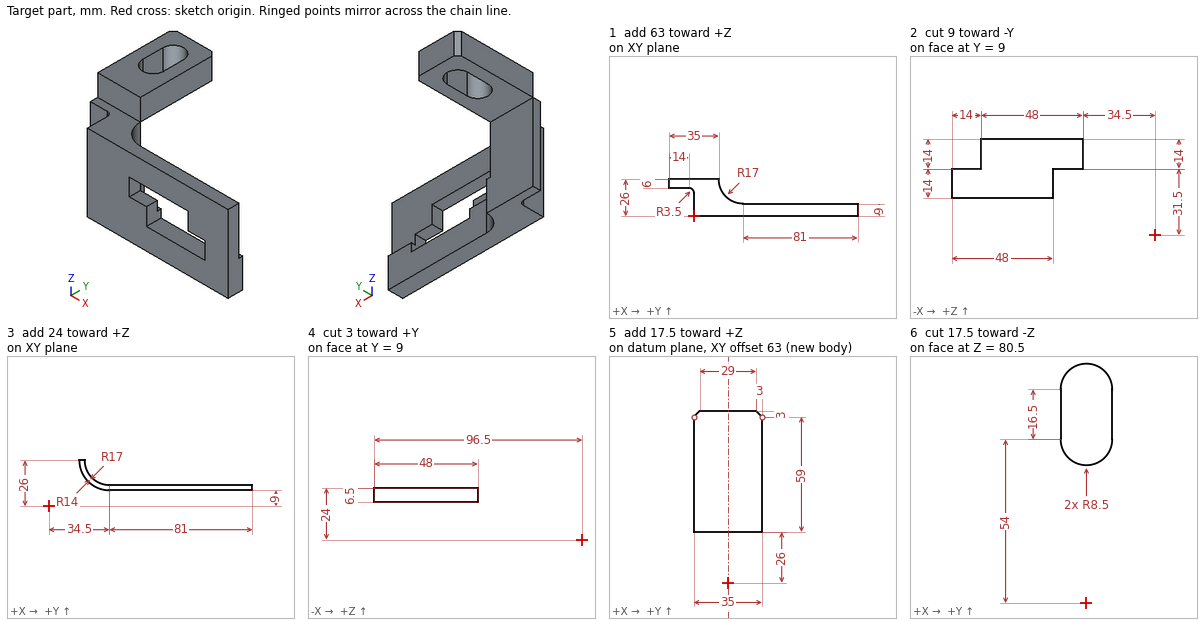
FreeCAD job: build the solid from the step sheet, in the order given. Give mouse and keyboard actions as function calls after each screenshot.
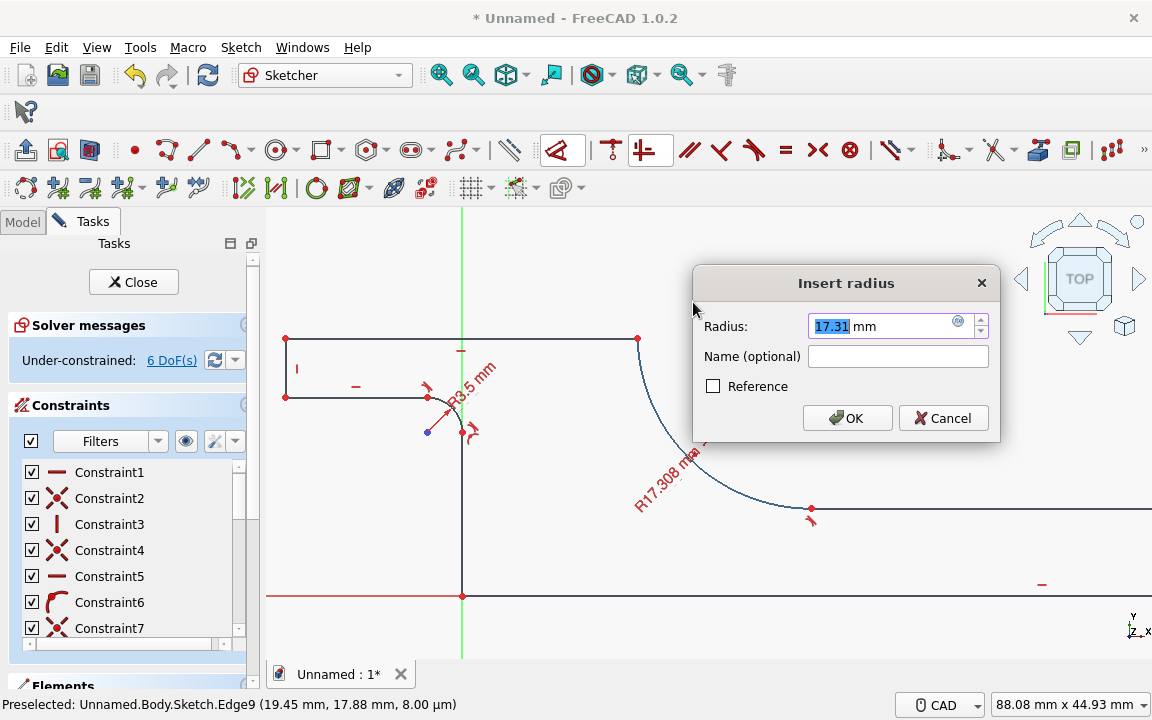
text(17)
key(Return)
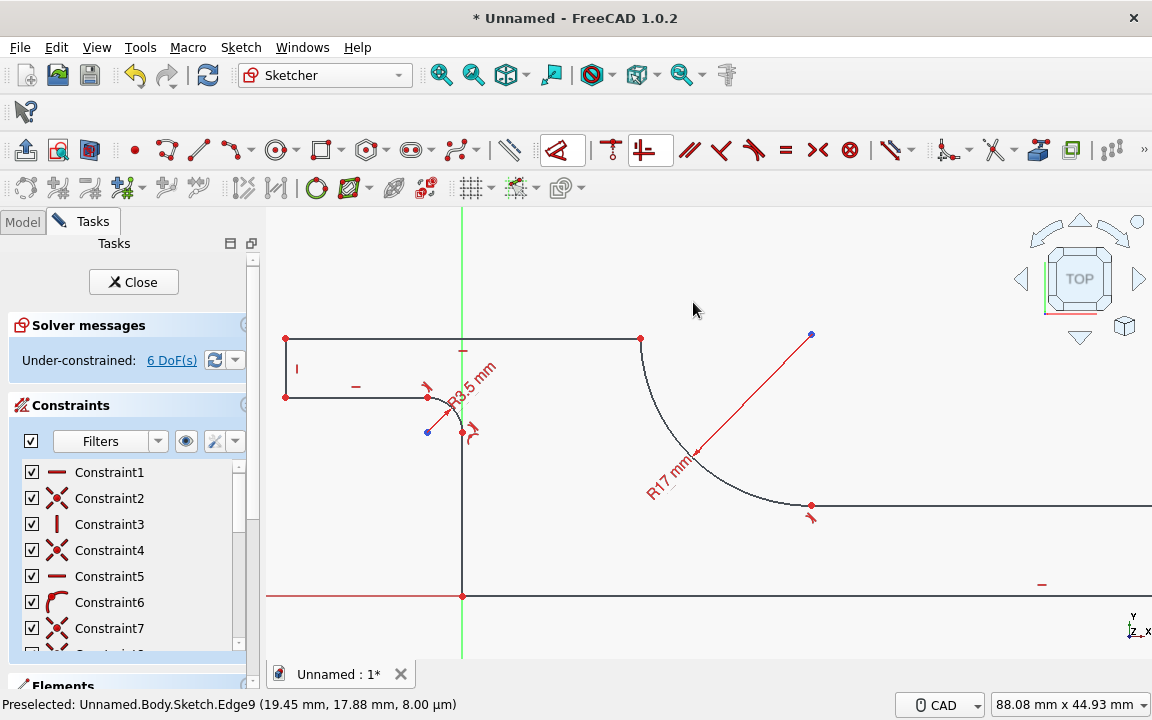
scroll(457, 414, down, 5)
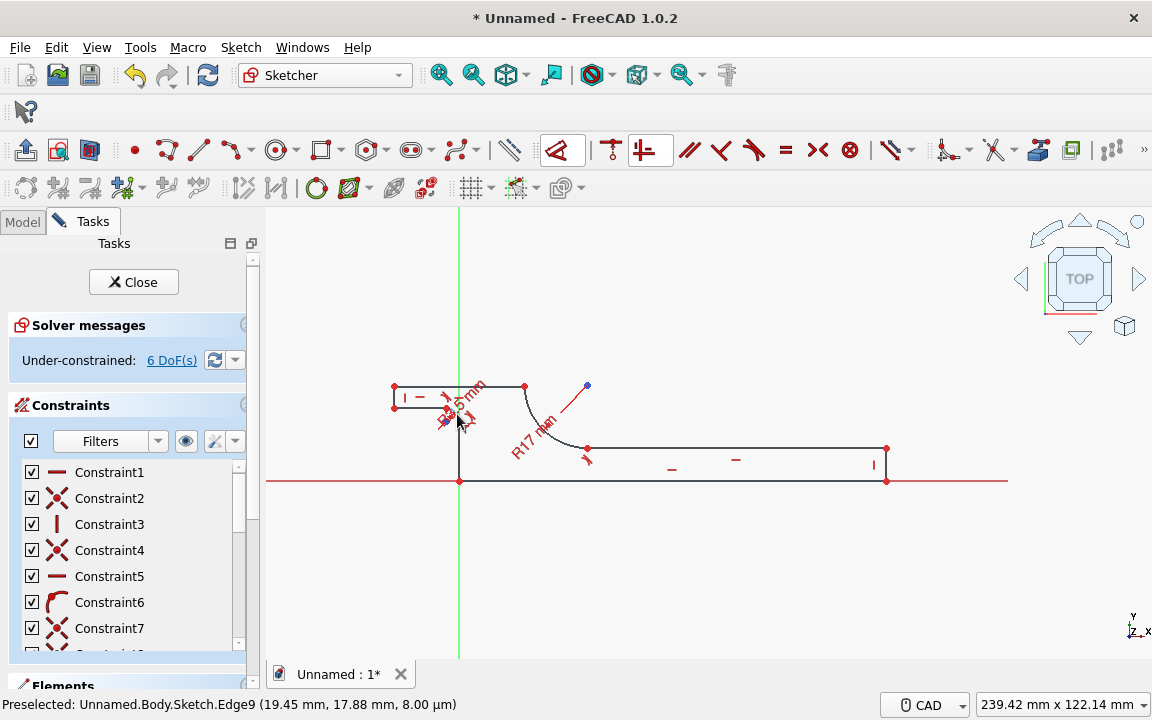
scroll(394, 393, up, 4)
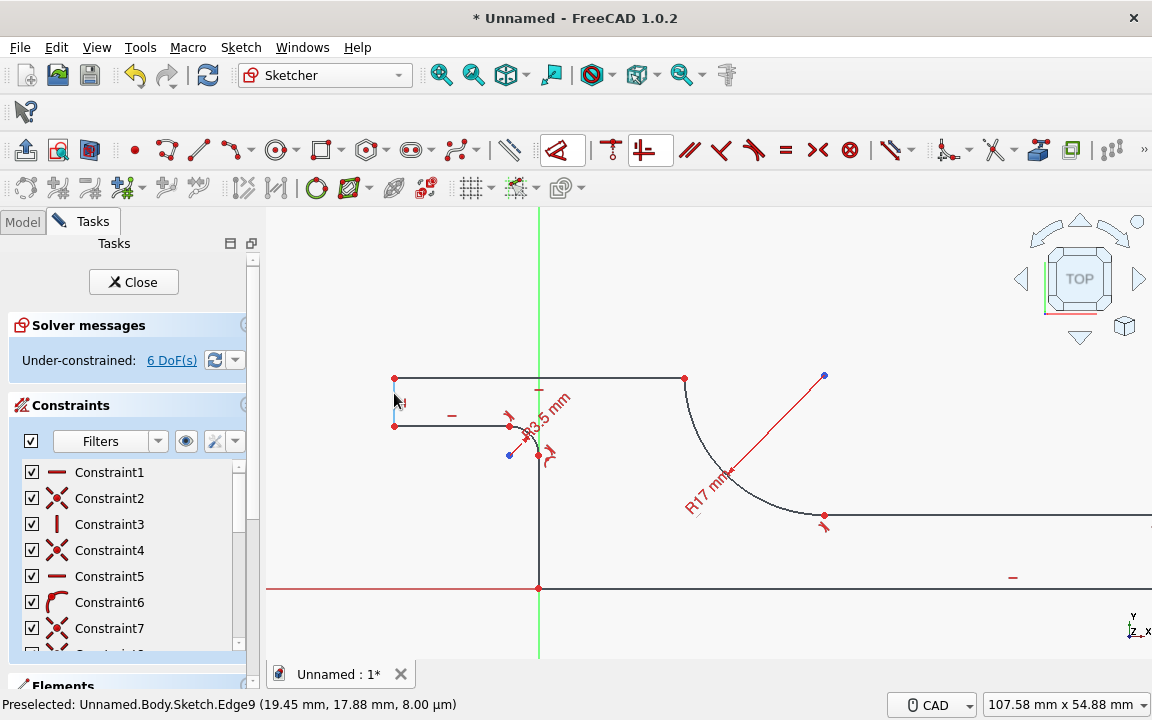
click(394, 393)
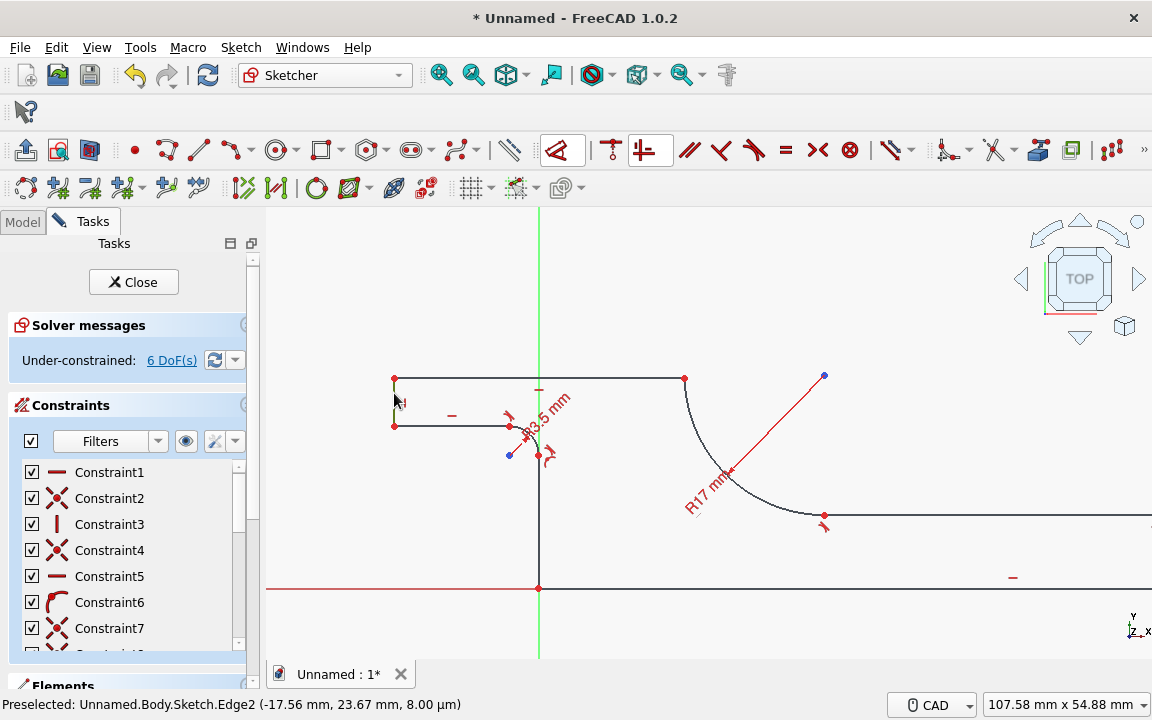
key(i)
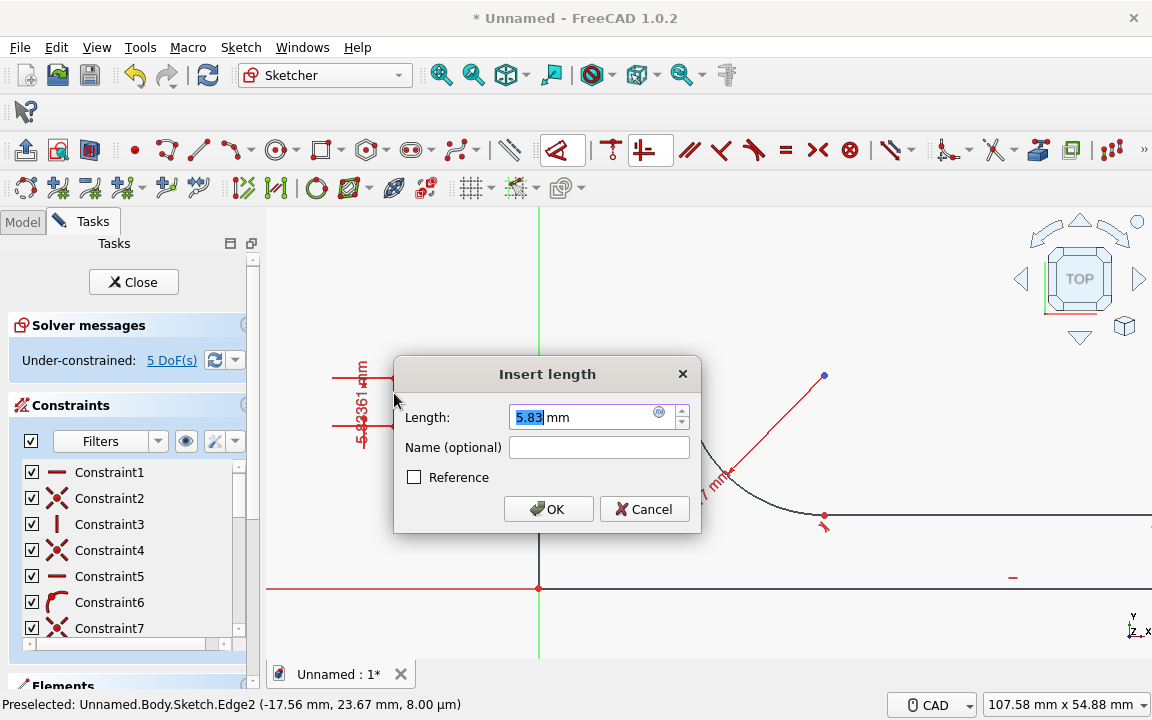
text(6)
key(Return)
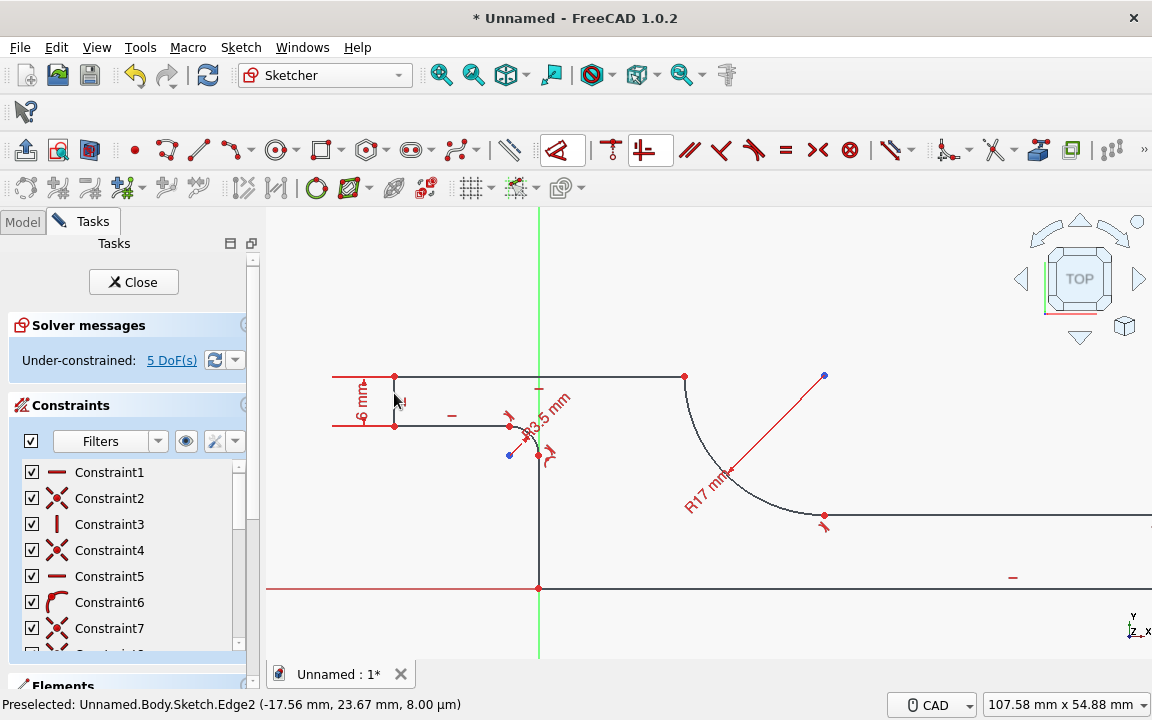
scroll(394, 393, down, 4)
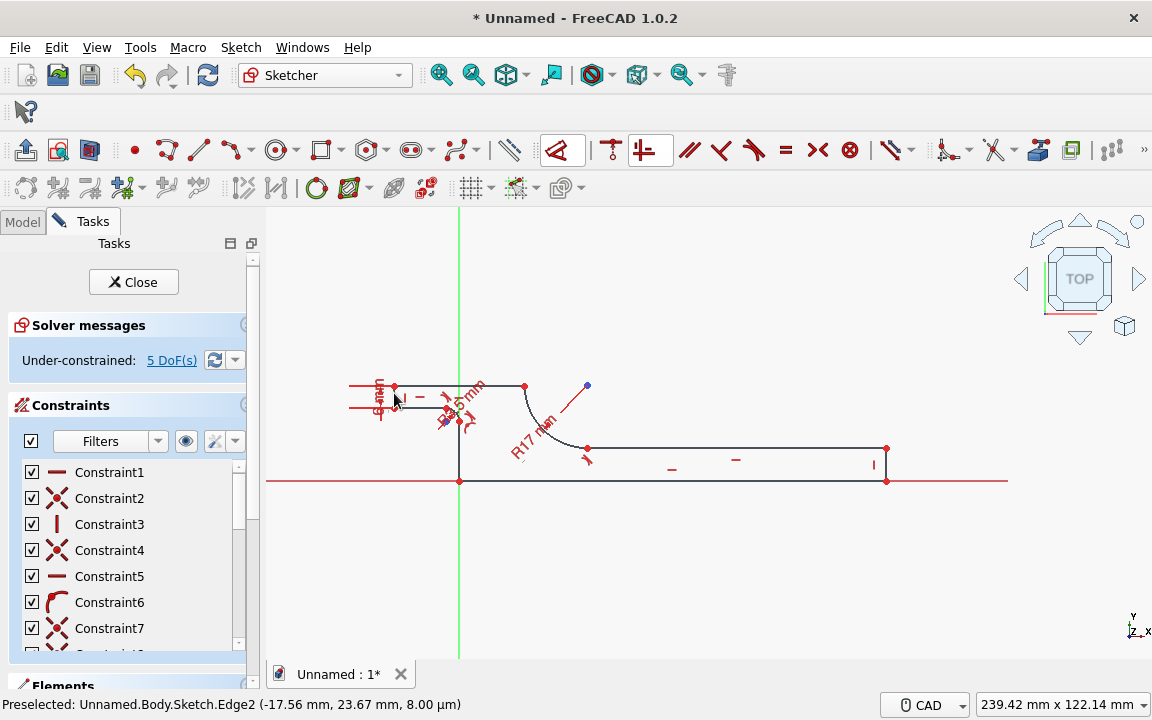
scroll(886, 471, up, 2)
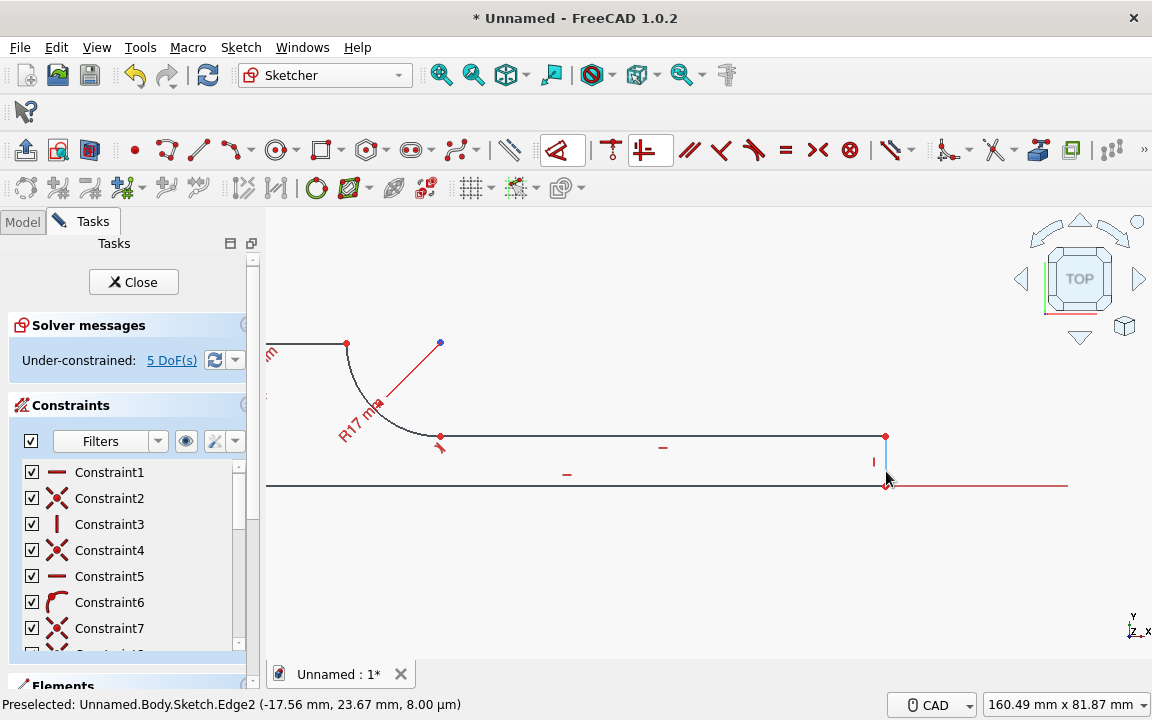
click(886, 471)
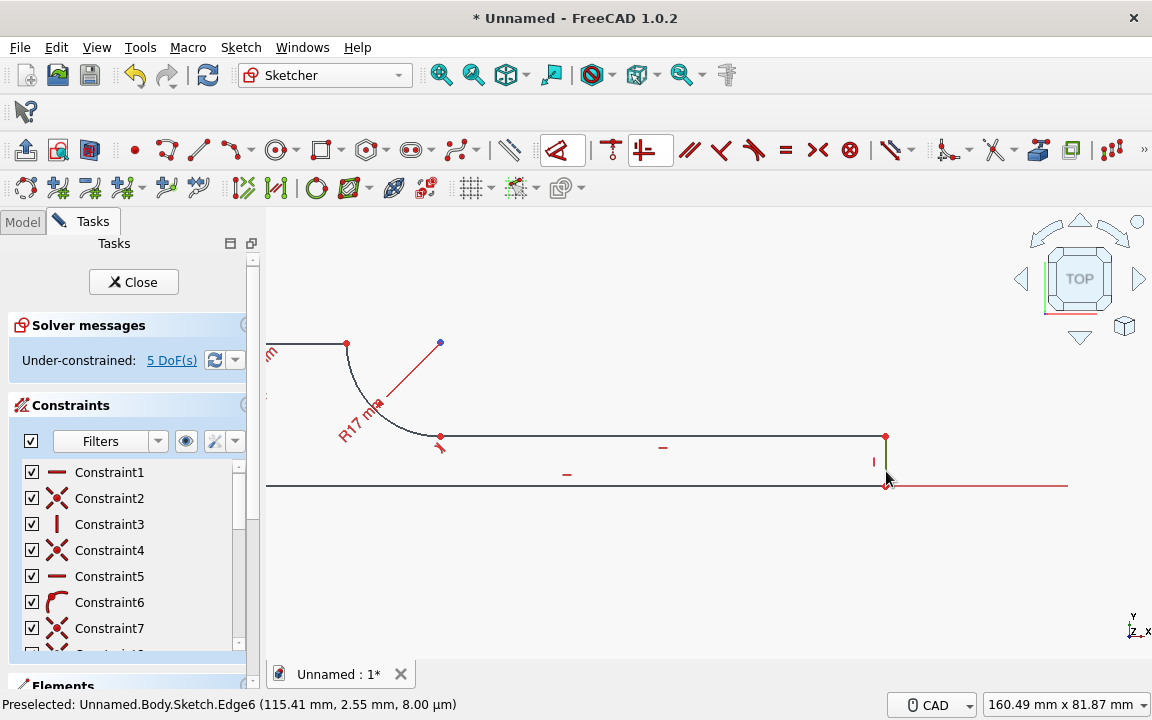
key(i)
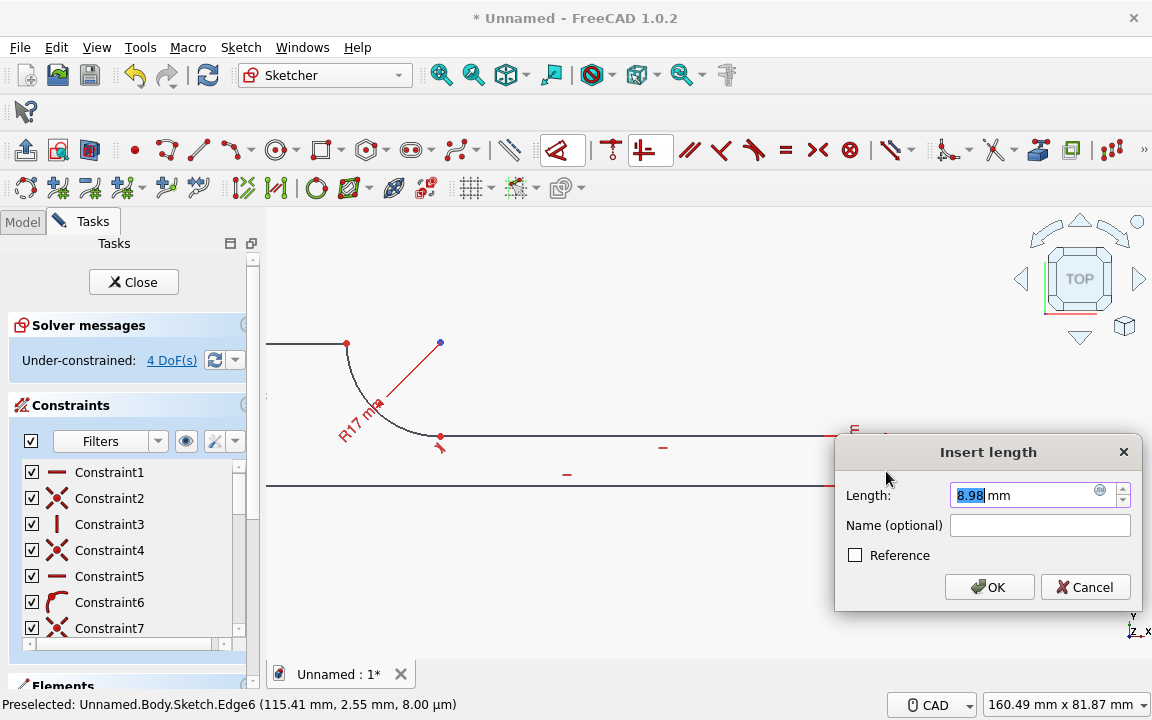
text(9)
key(Return)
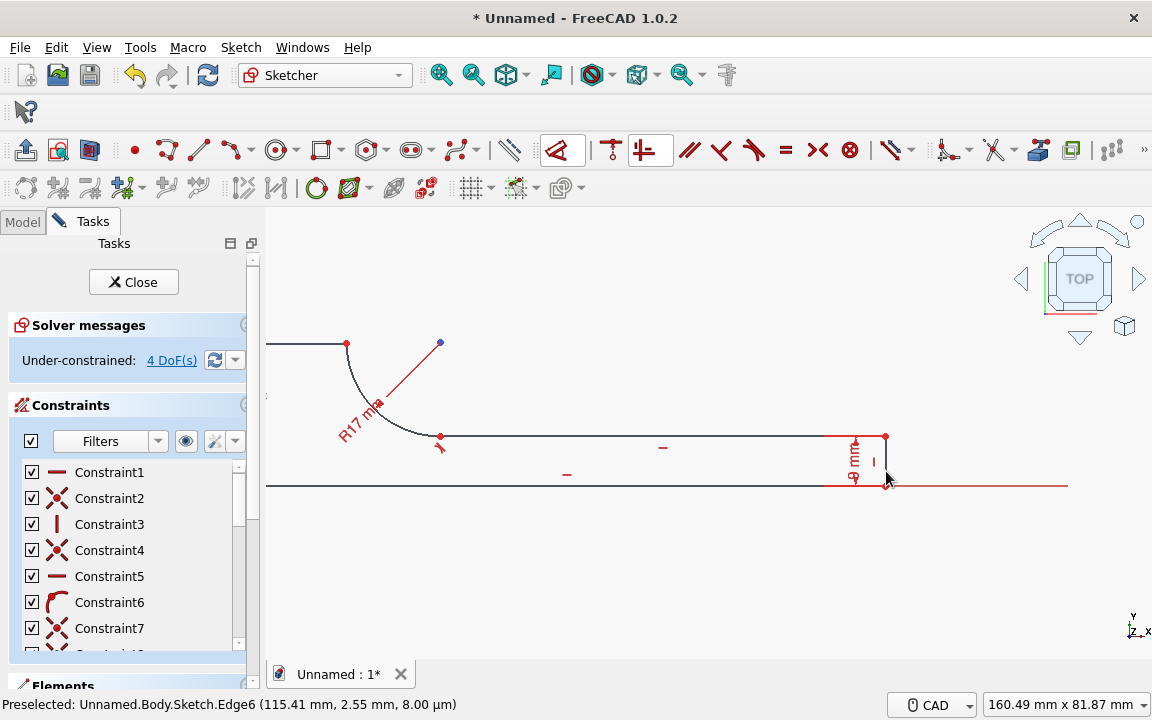
click(308, 344)